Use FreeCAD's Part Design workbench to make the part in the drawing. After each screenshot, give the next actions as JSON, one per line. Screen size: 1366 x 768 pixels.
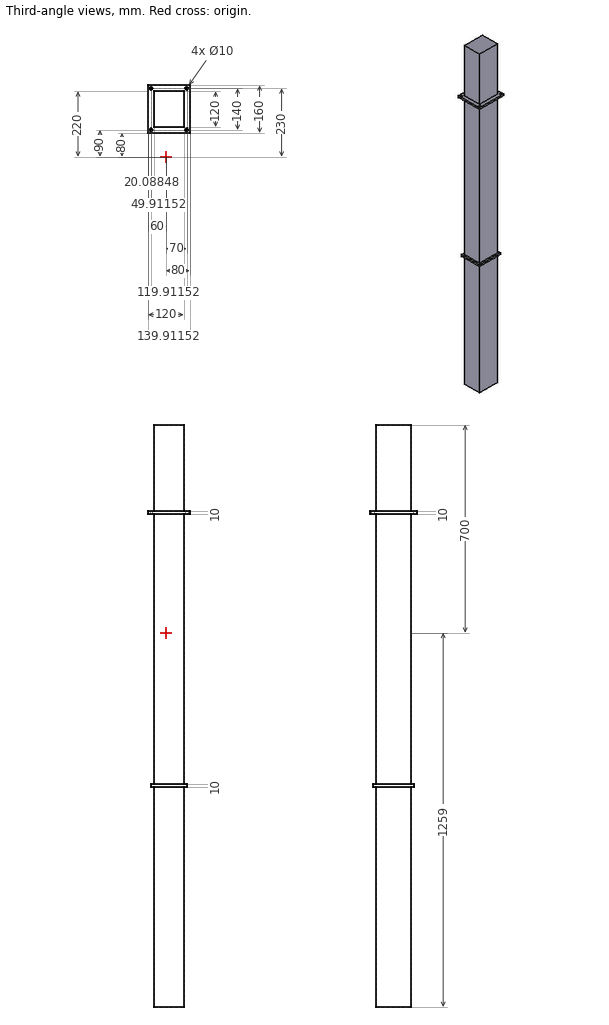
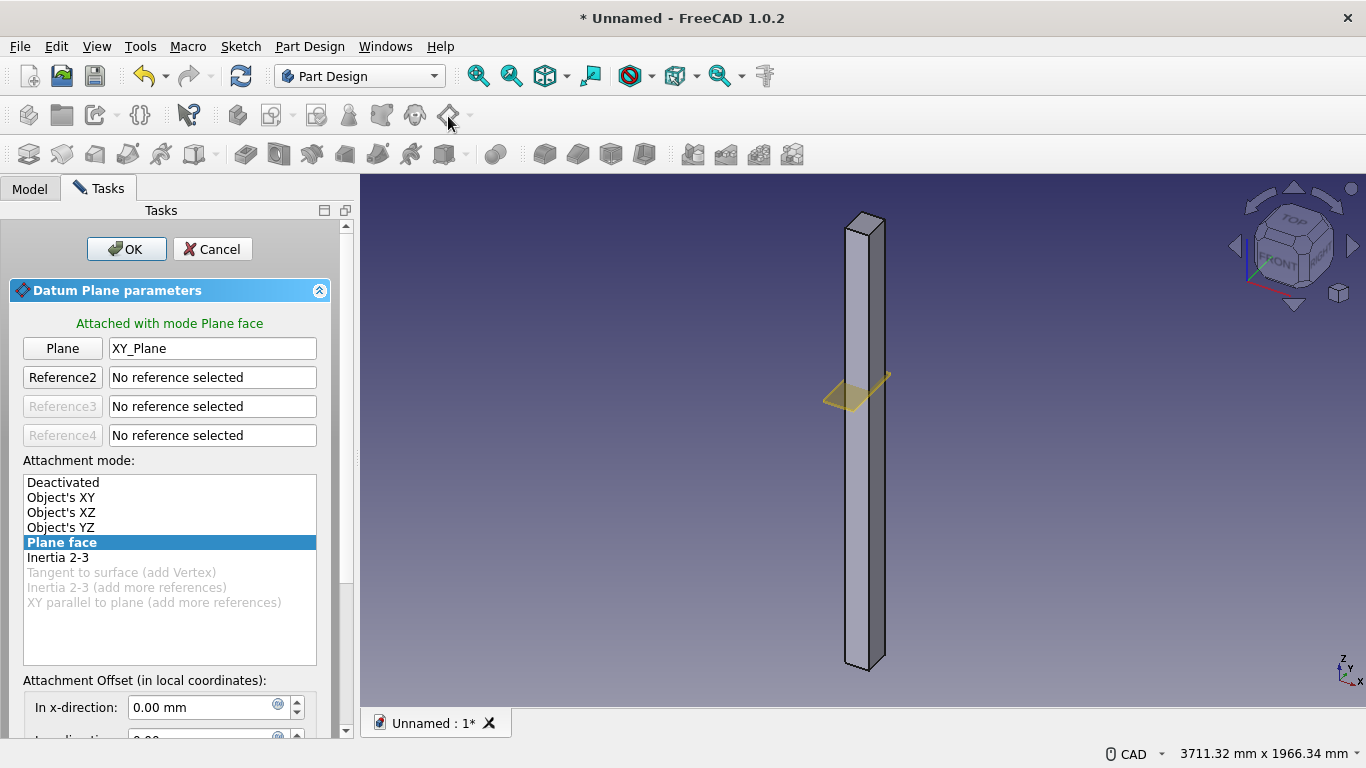
{"action": "scroll", "coordinate": [346, 479], "scroll_direction": "down", "scroll_amount": 2}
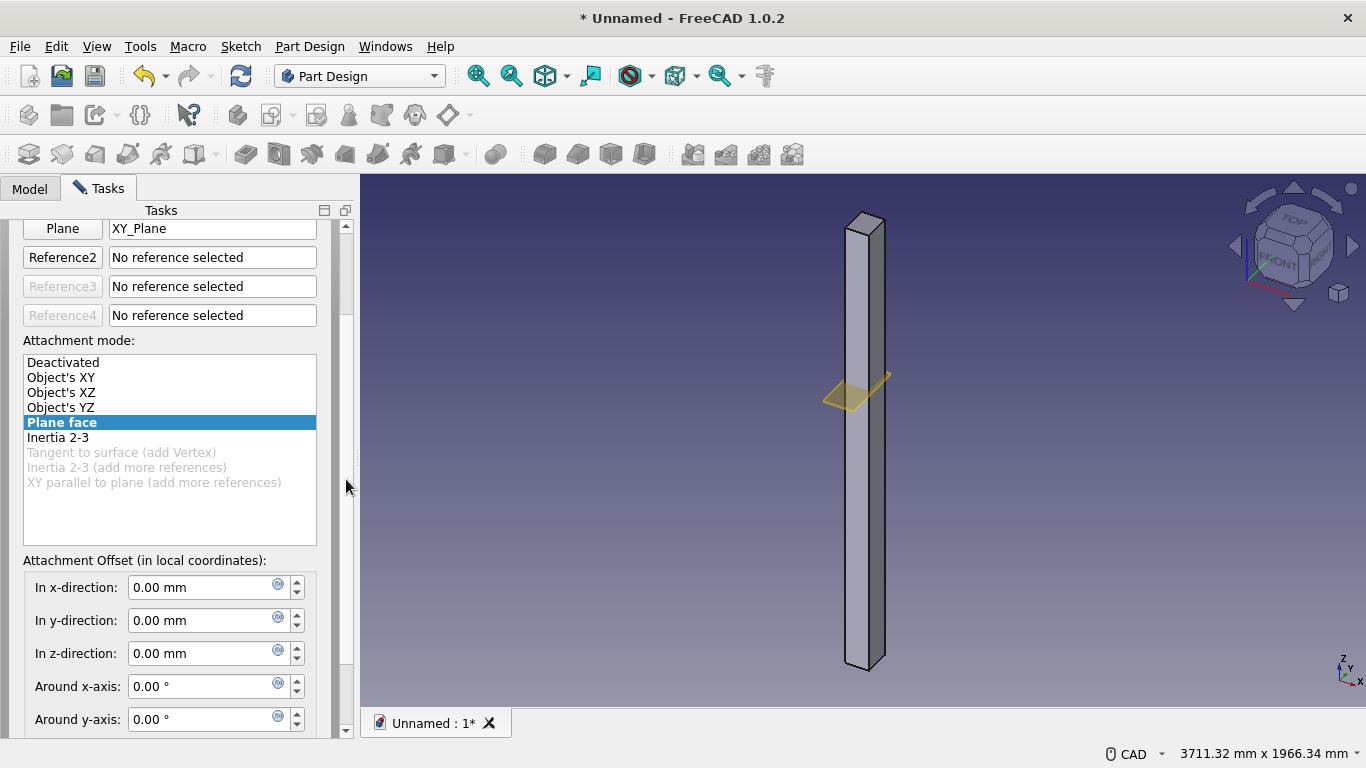
{"action": "triple_click", "coordinate": [210, 654]}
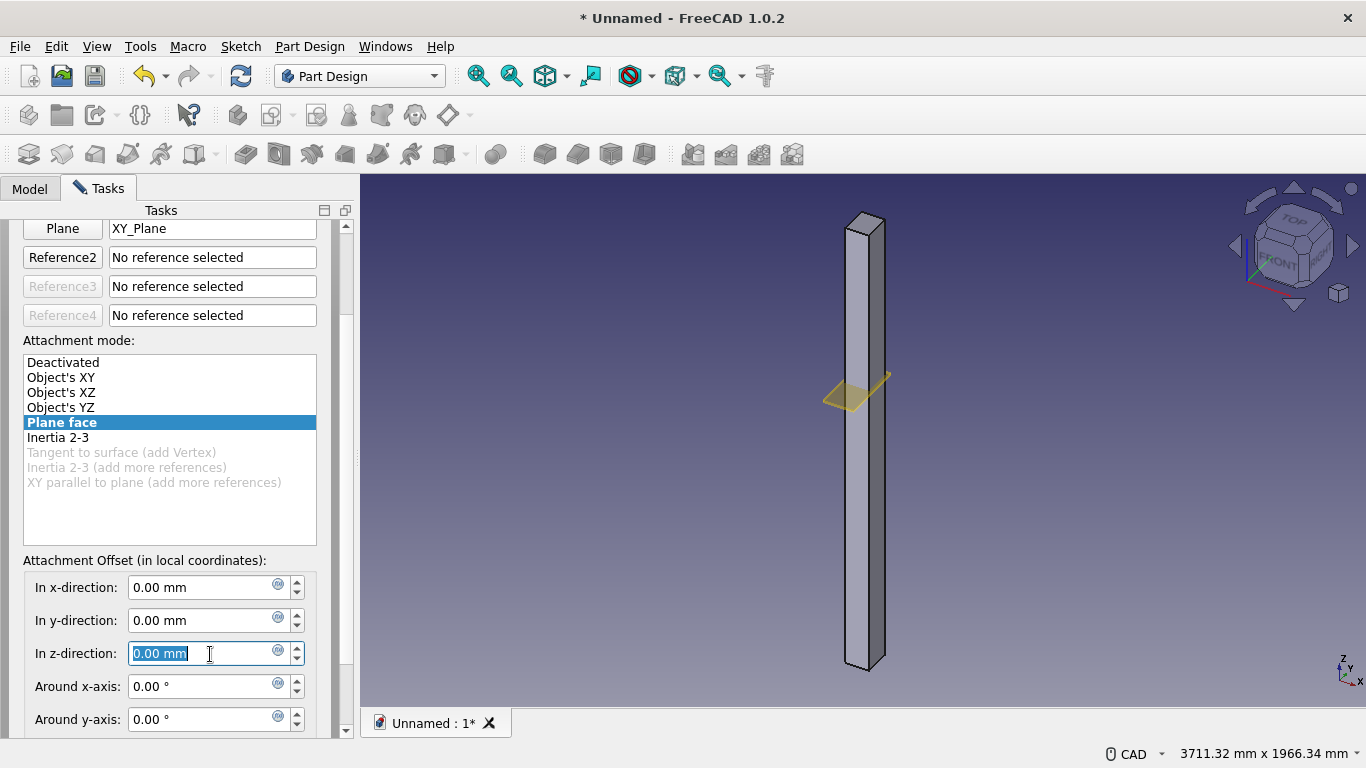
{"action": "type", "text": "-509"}
{"action": "key", "text": "Tab"}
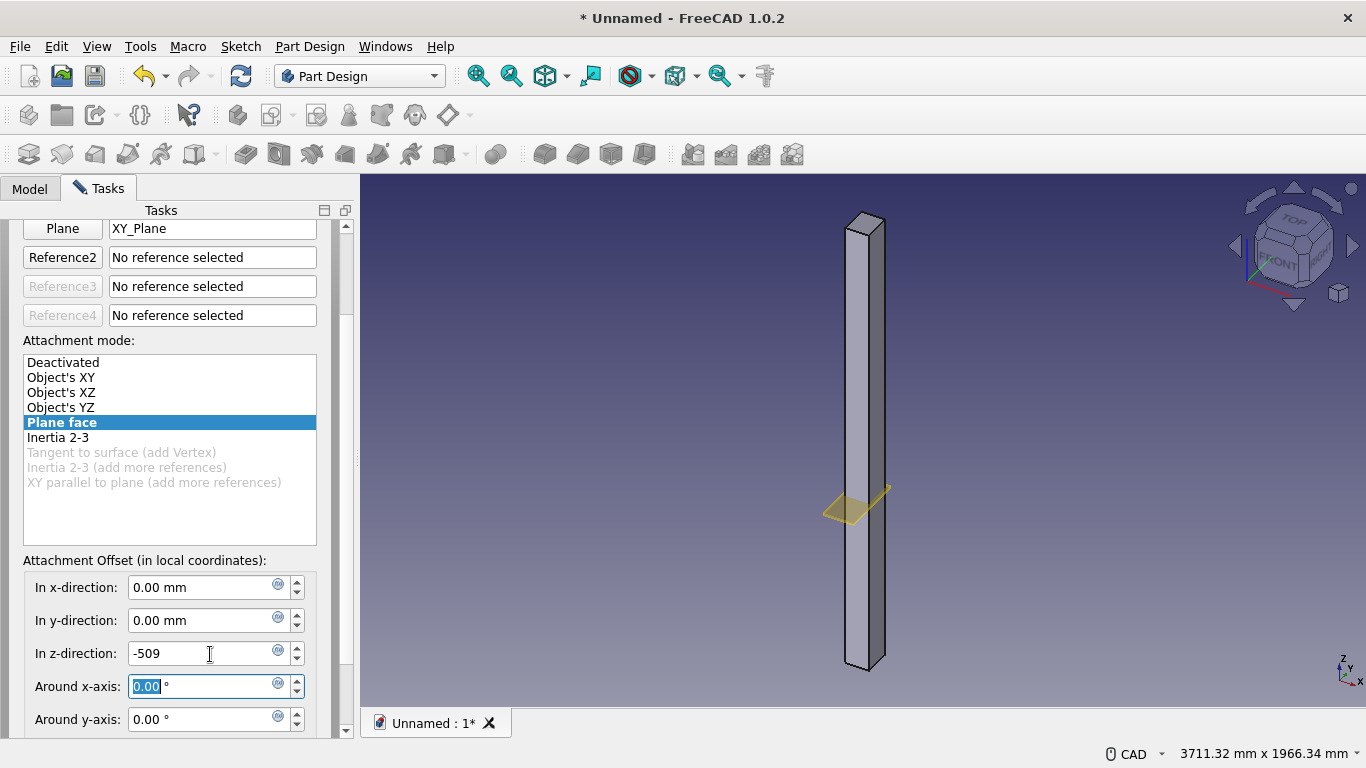
{"action": "scroll", "coordinate": [346, 479], "scroll_direction": "up", "scroll_amount": 3}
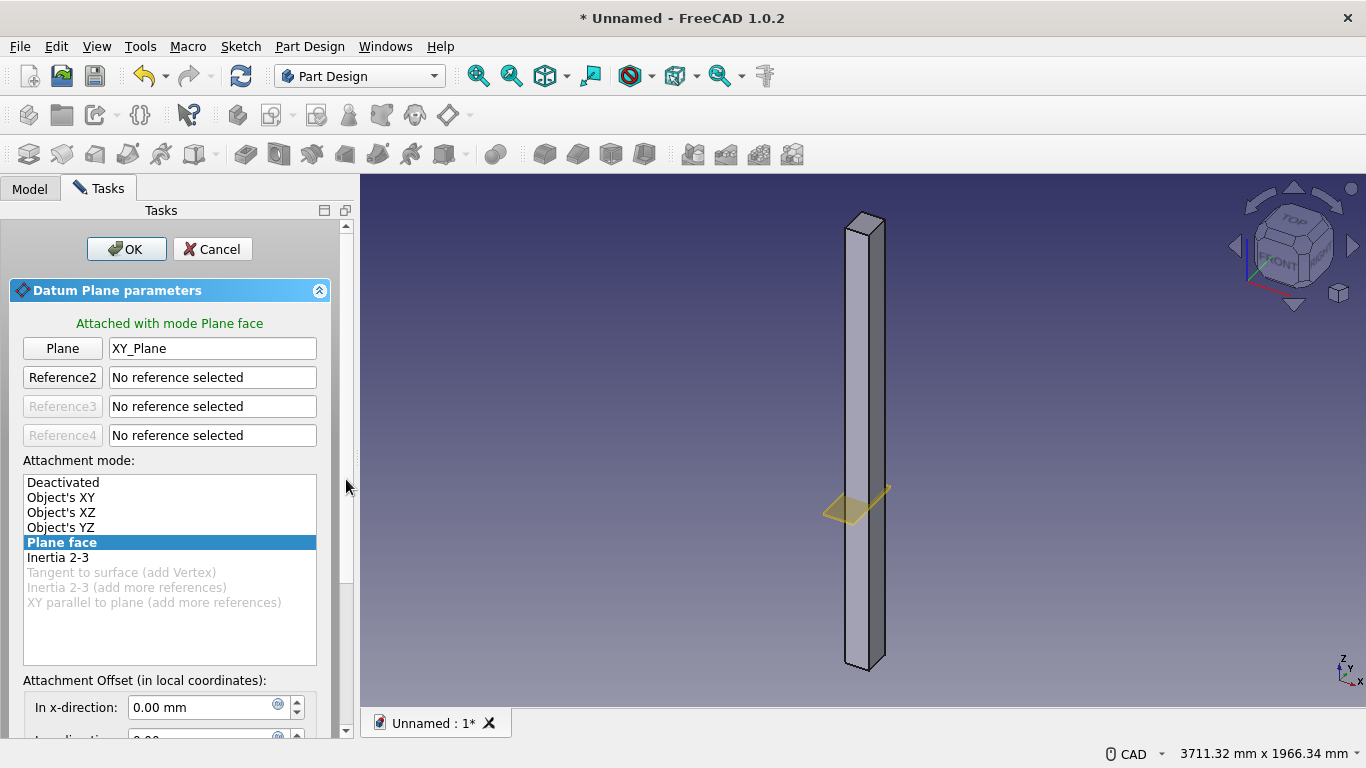
{"action": "left_click", "coordinate": [127, 249]}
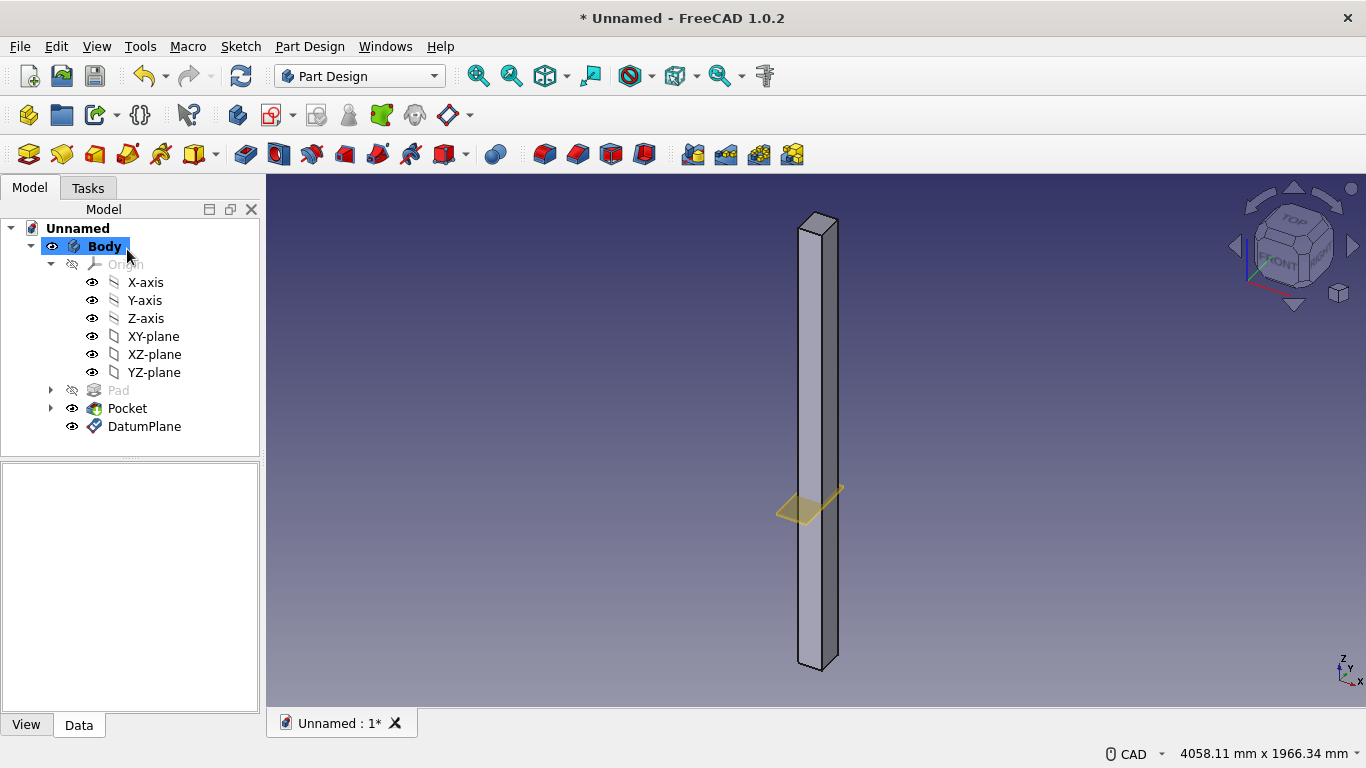
{"action": "left_click", "coordinate": [117, 426]}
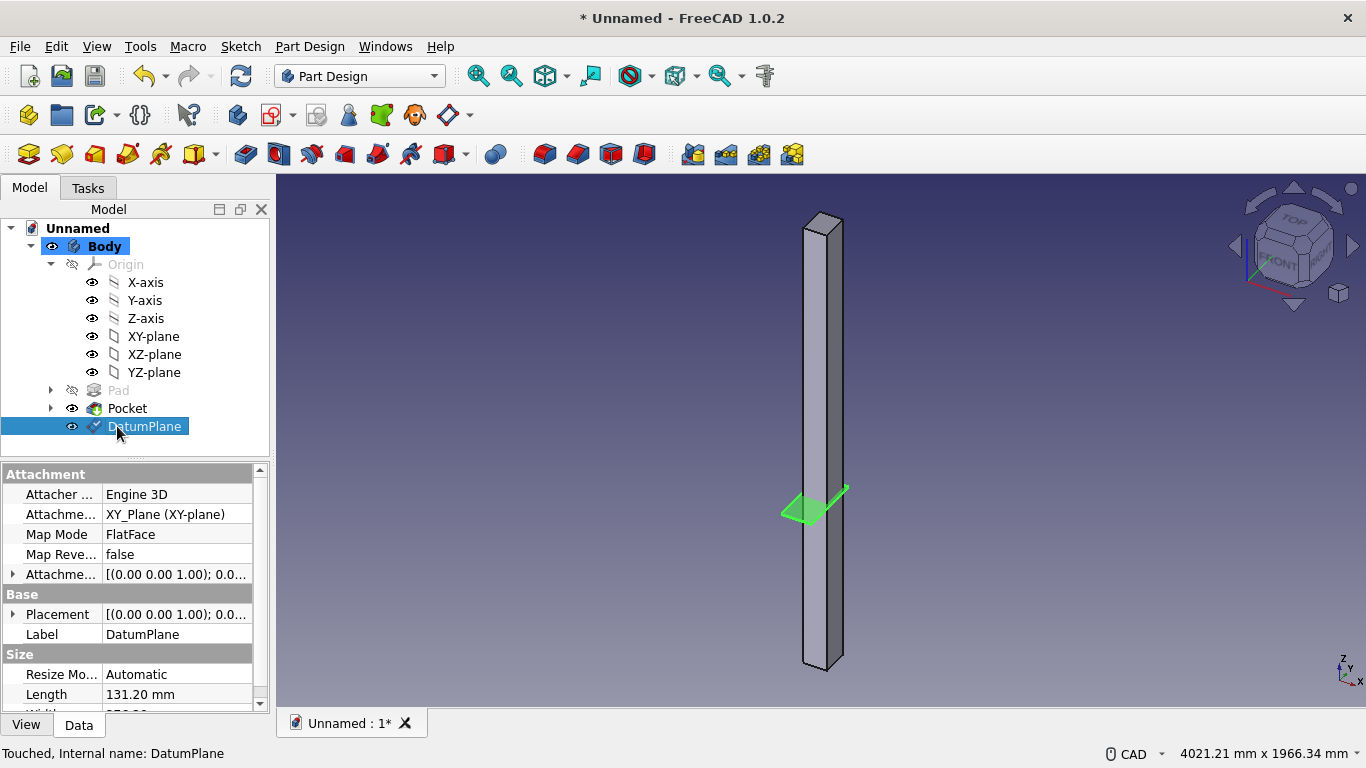
{"action": "left_click", "coordinate": [270, 116]}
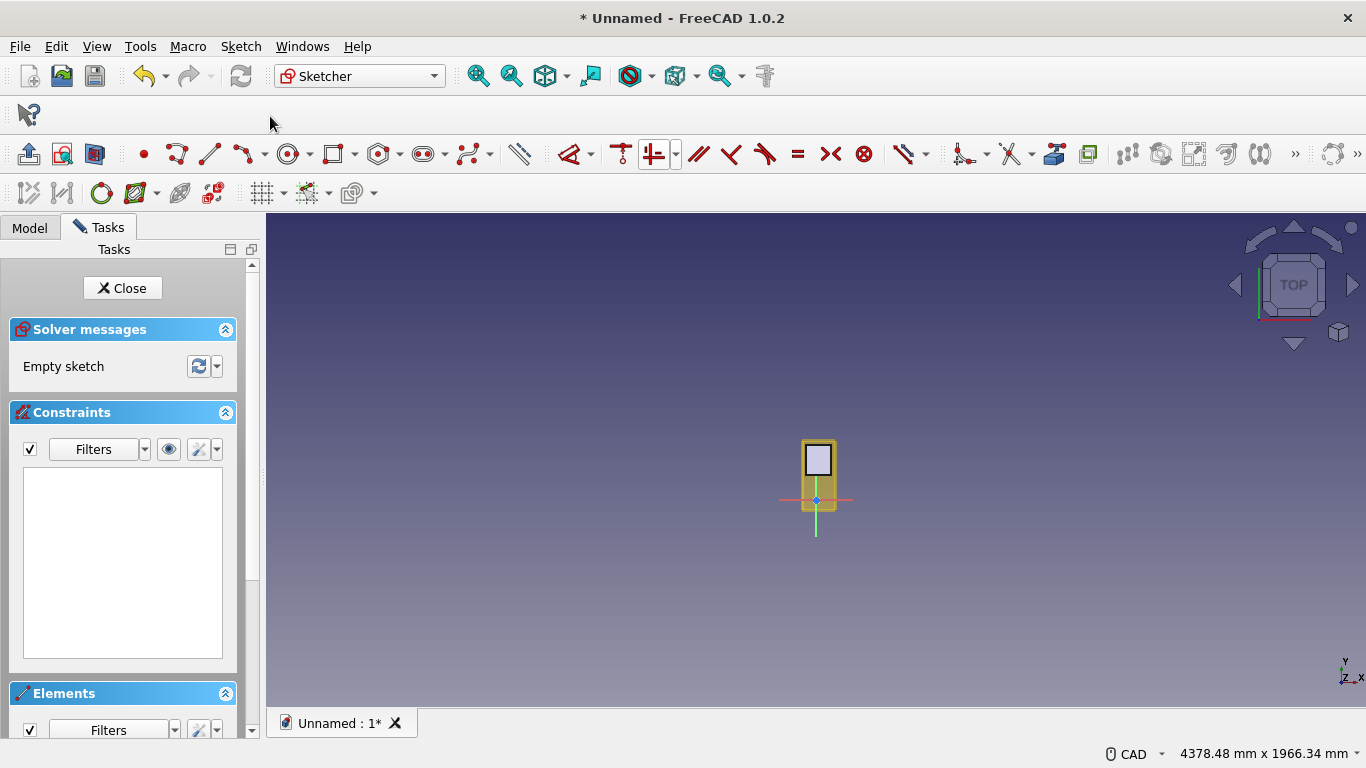
{"action": "key", "text": "q s"}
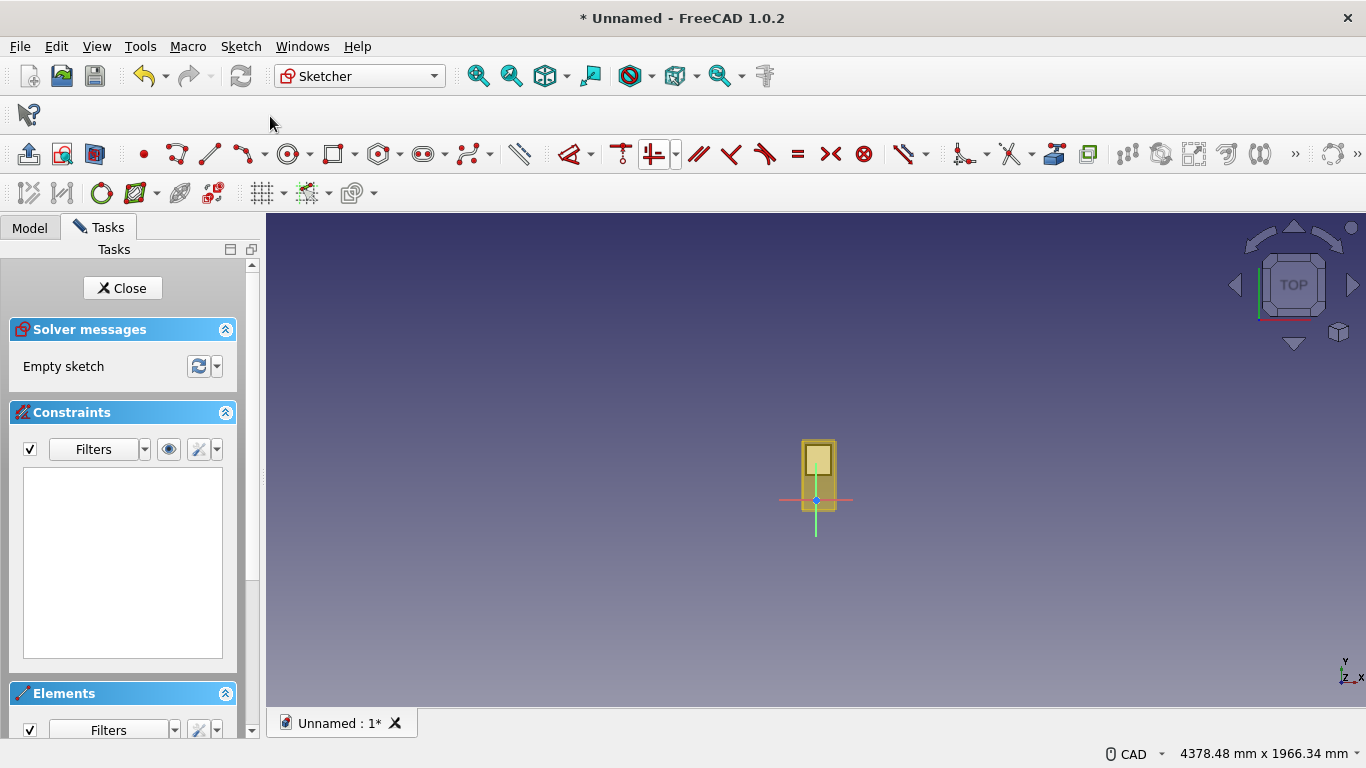
{"action": "scroll", "coordinate": [836, 474], "scroll_direction": "up", "scroll_amount": 8}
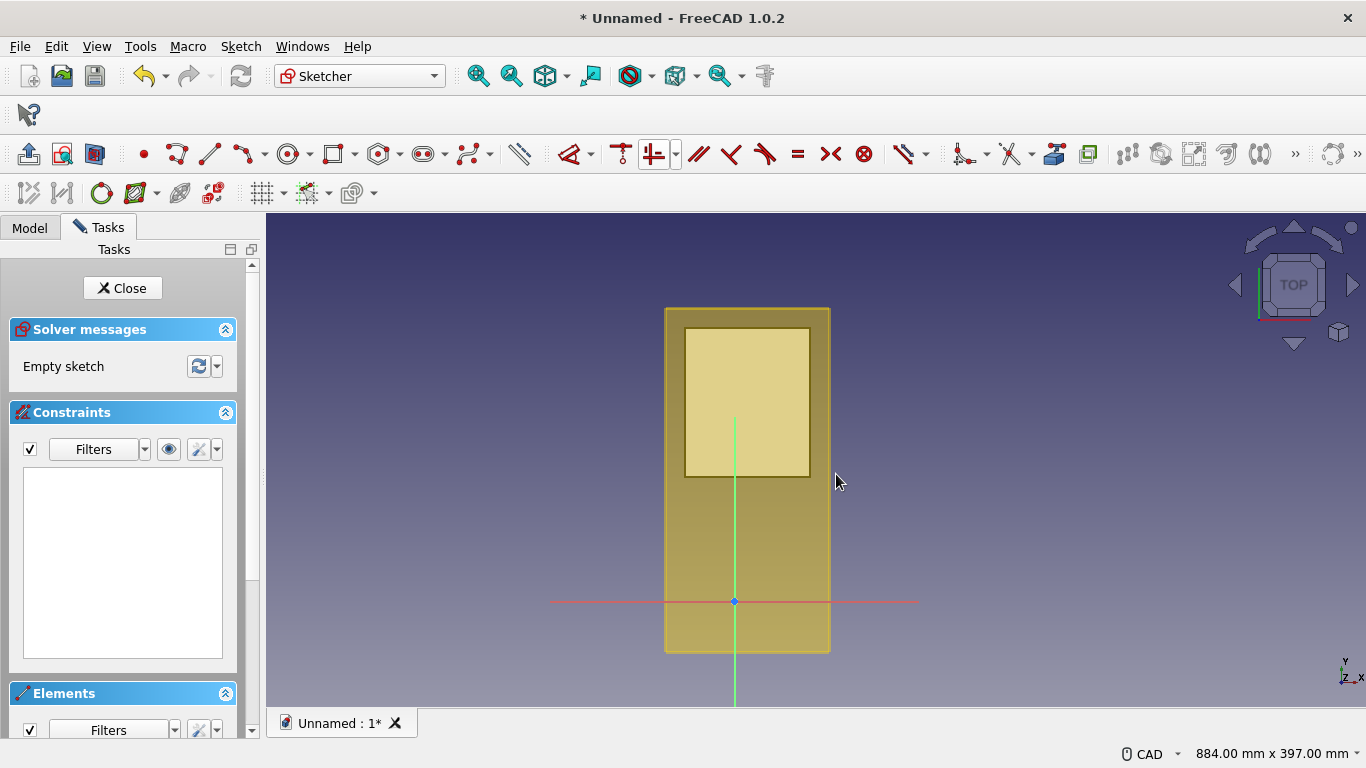
{"action": "left_click", "coordinate": [332, 154]}